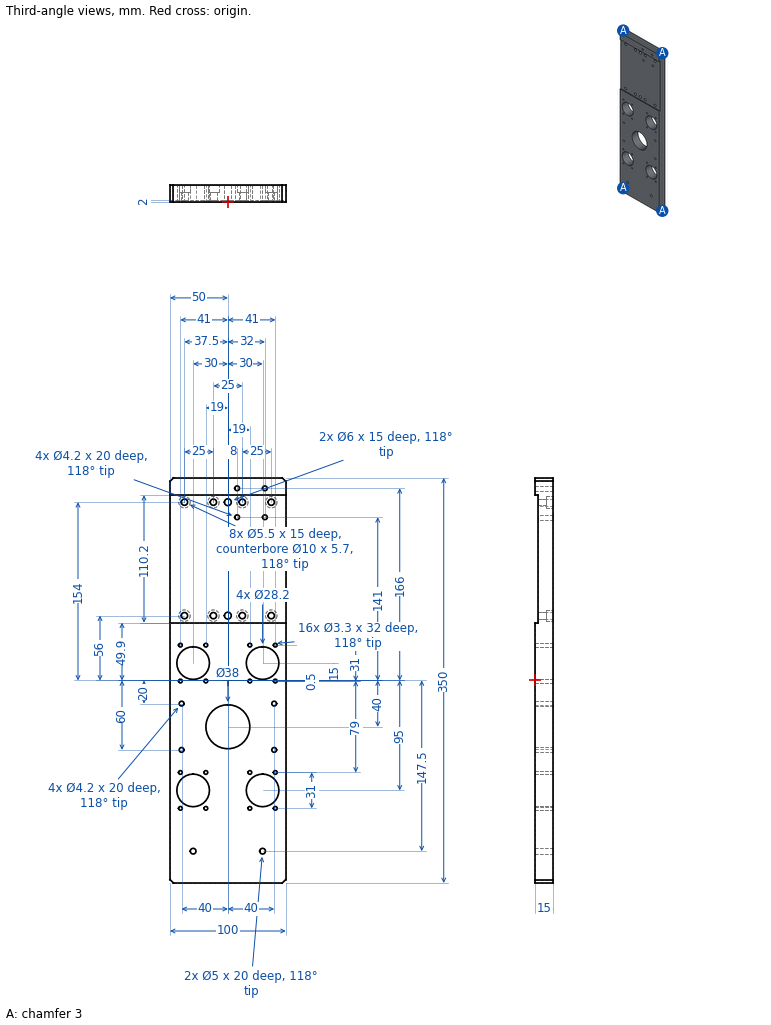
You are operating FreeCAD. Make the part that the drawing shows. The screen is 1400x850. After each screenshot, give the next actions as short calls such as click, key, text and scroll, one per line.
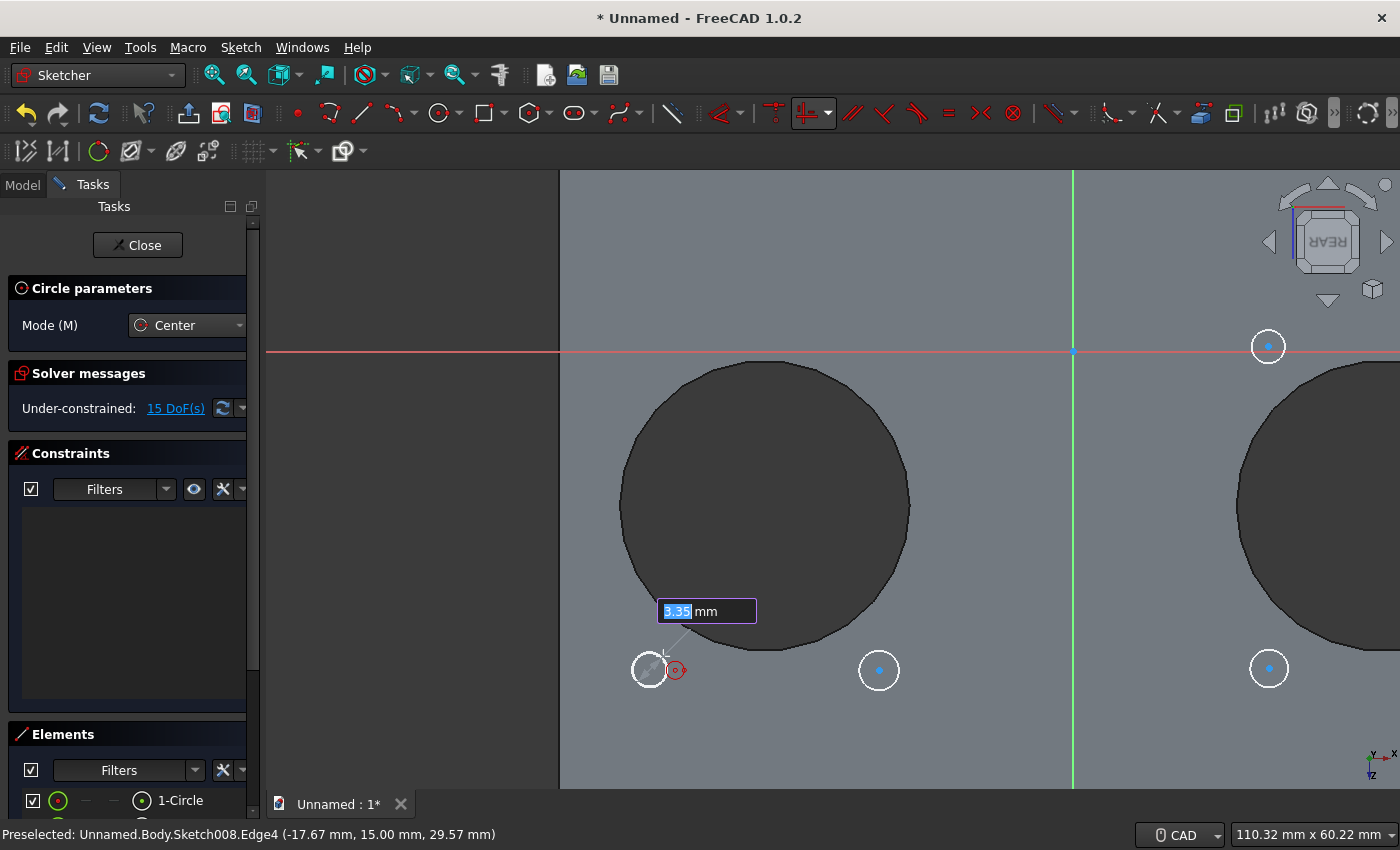
click(664, 653)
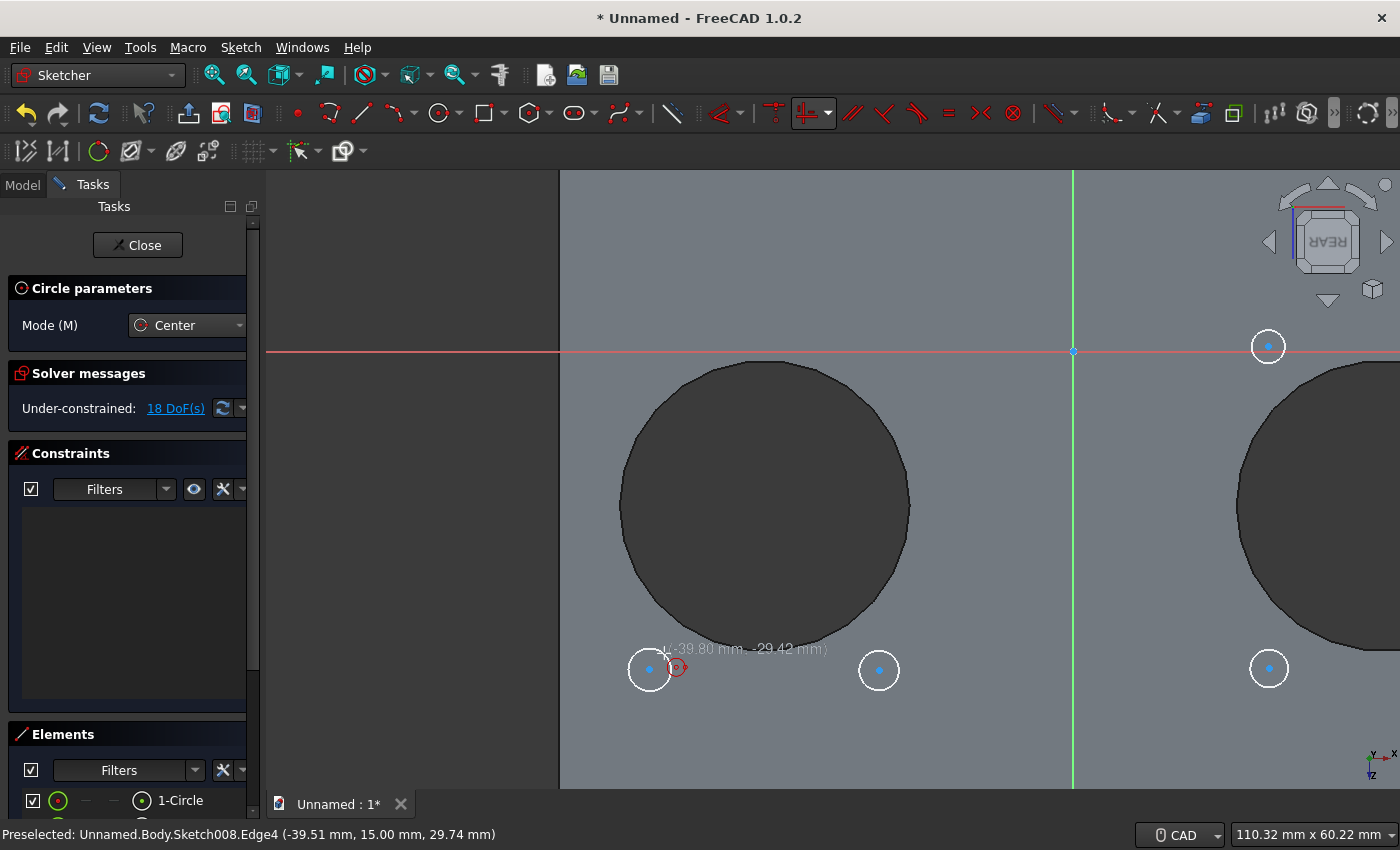
scroll(878, 346, up, 6)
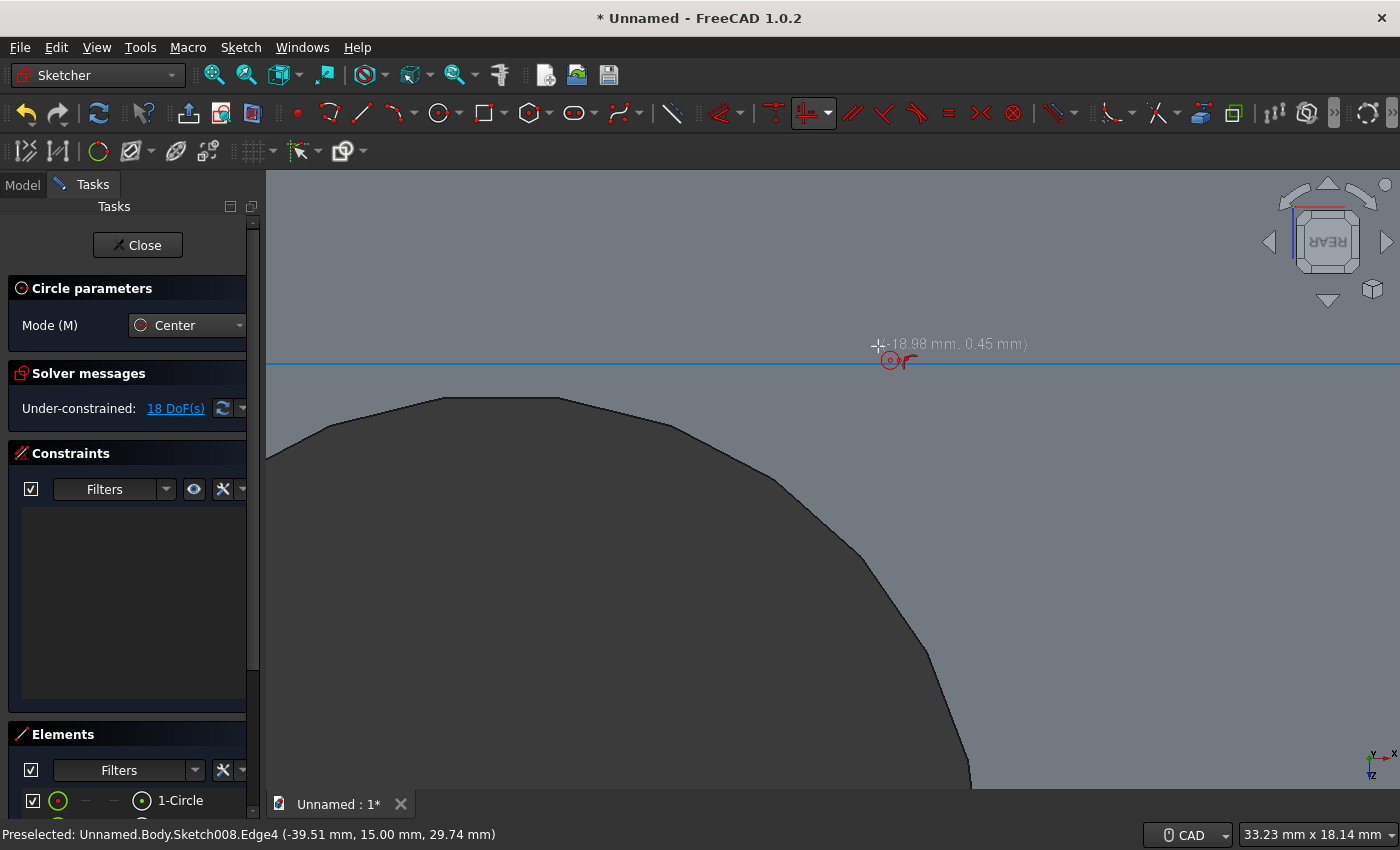
click(876, 347)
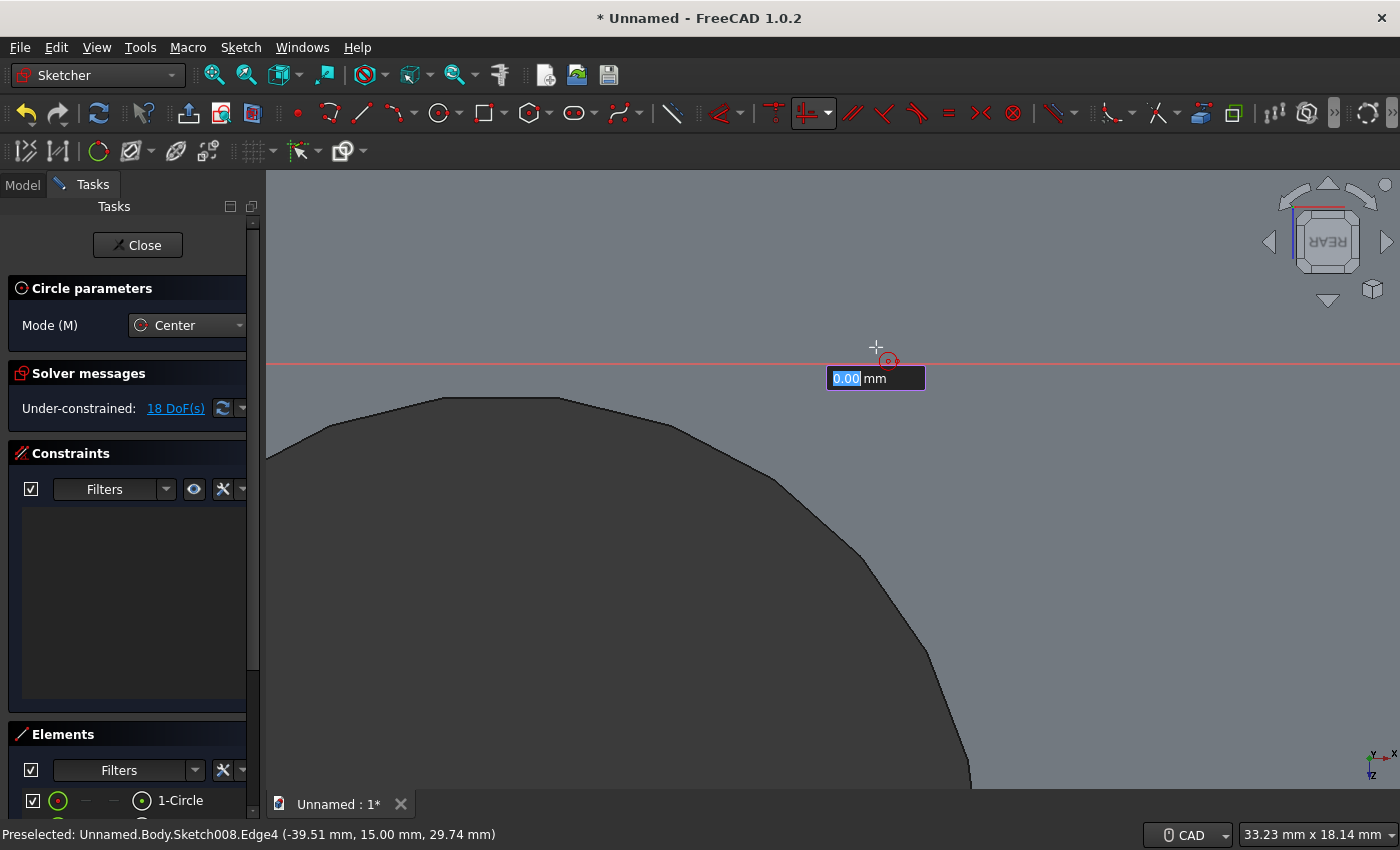
scroll(704, 598, down, 13)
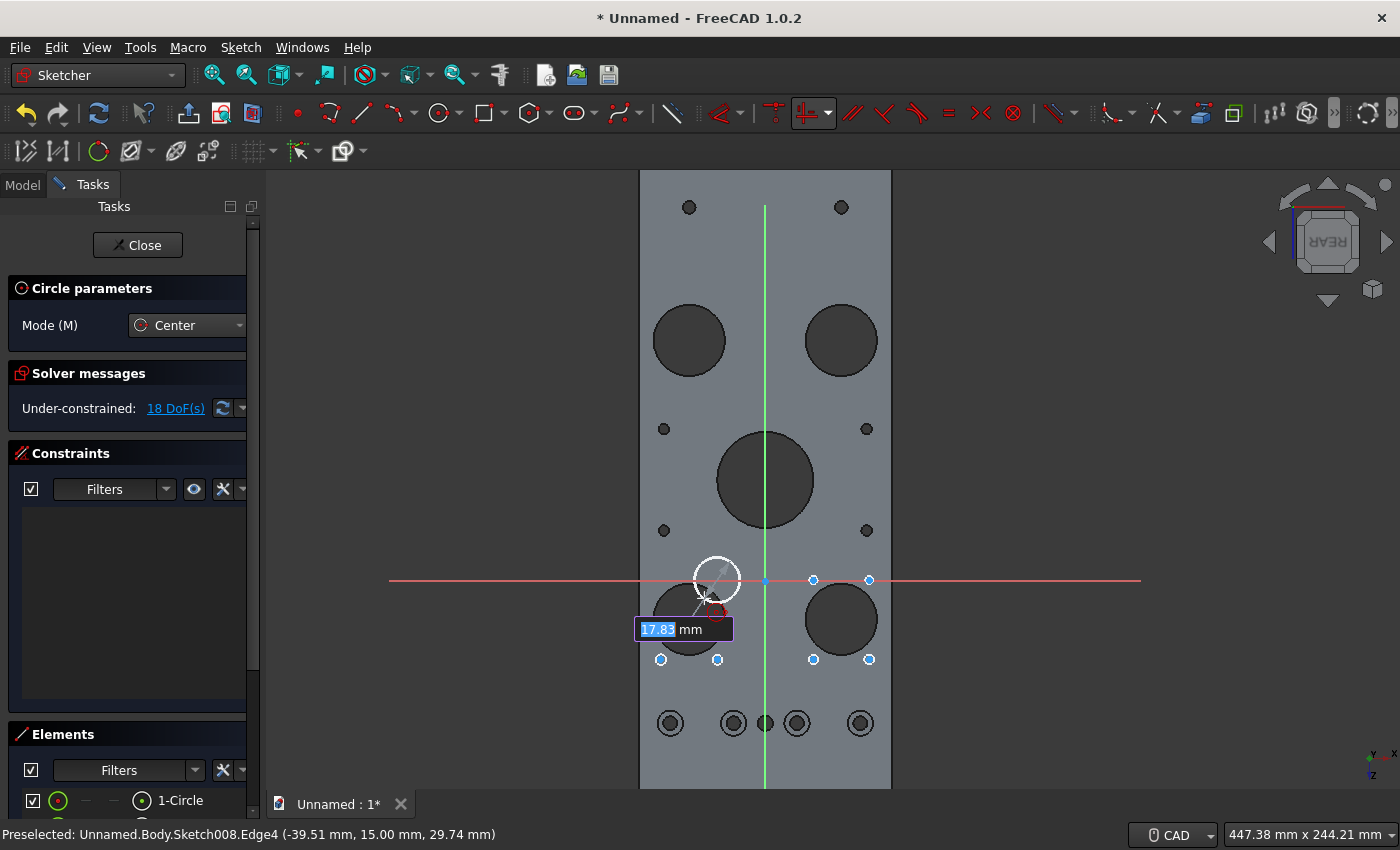
scroll(720, 577, up, 7)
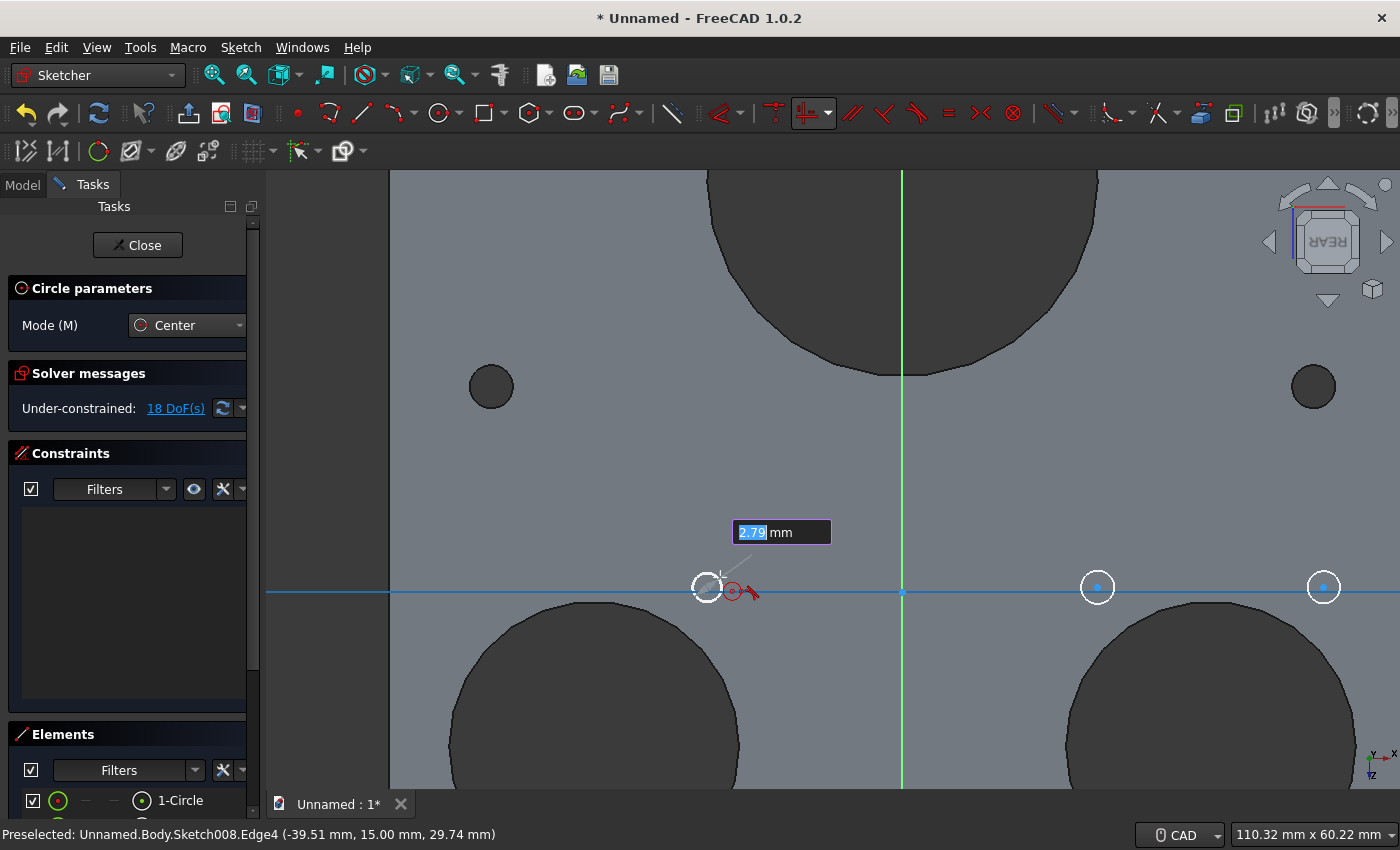
click(719, 575)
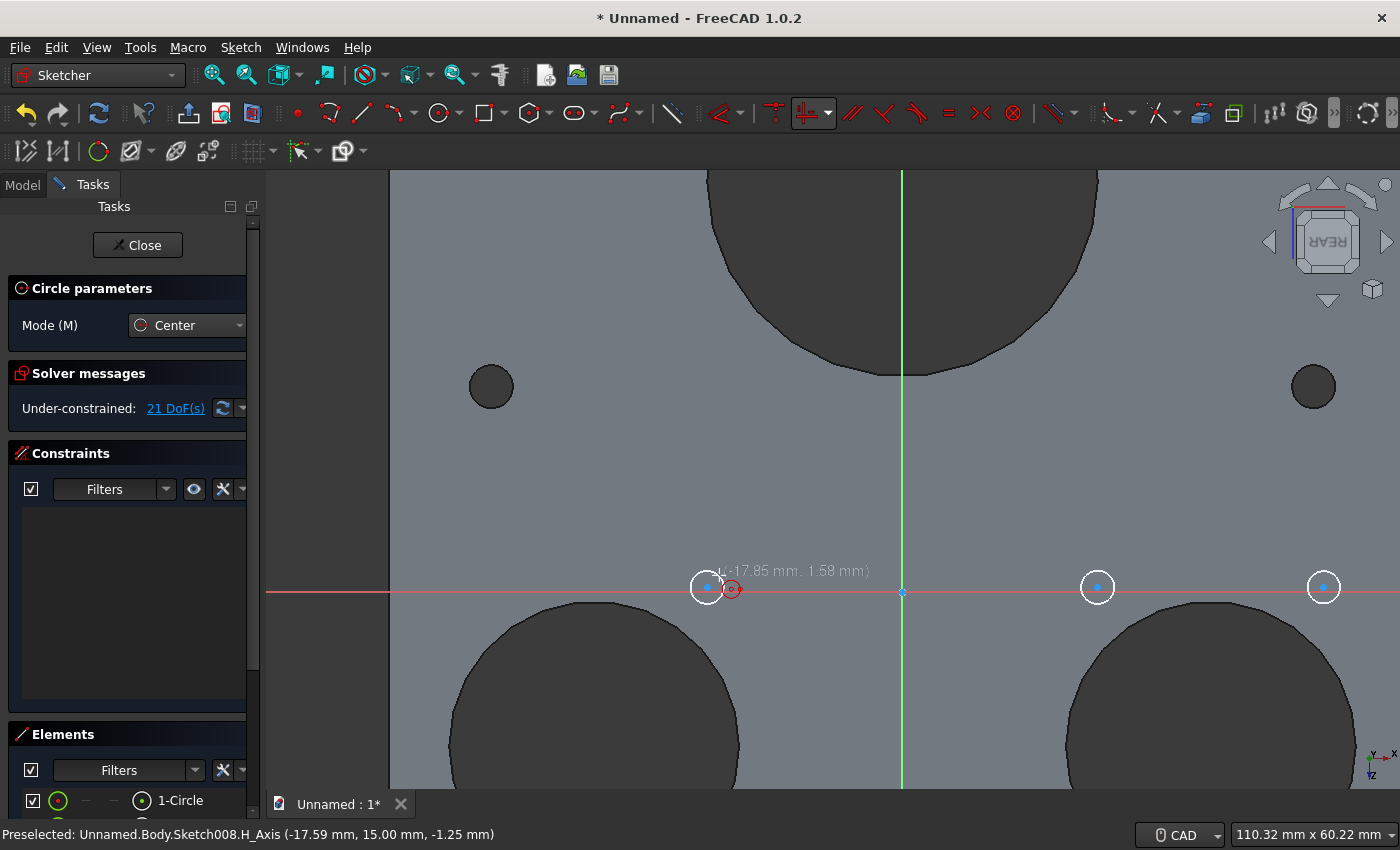
scroll(481, 587, up, 6)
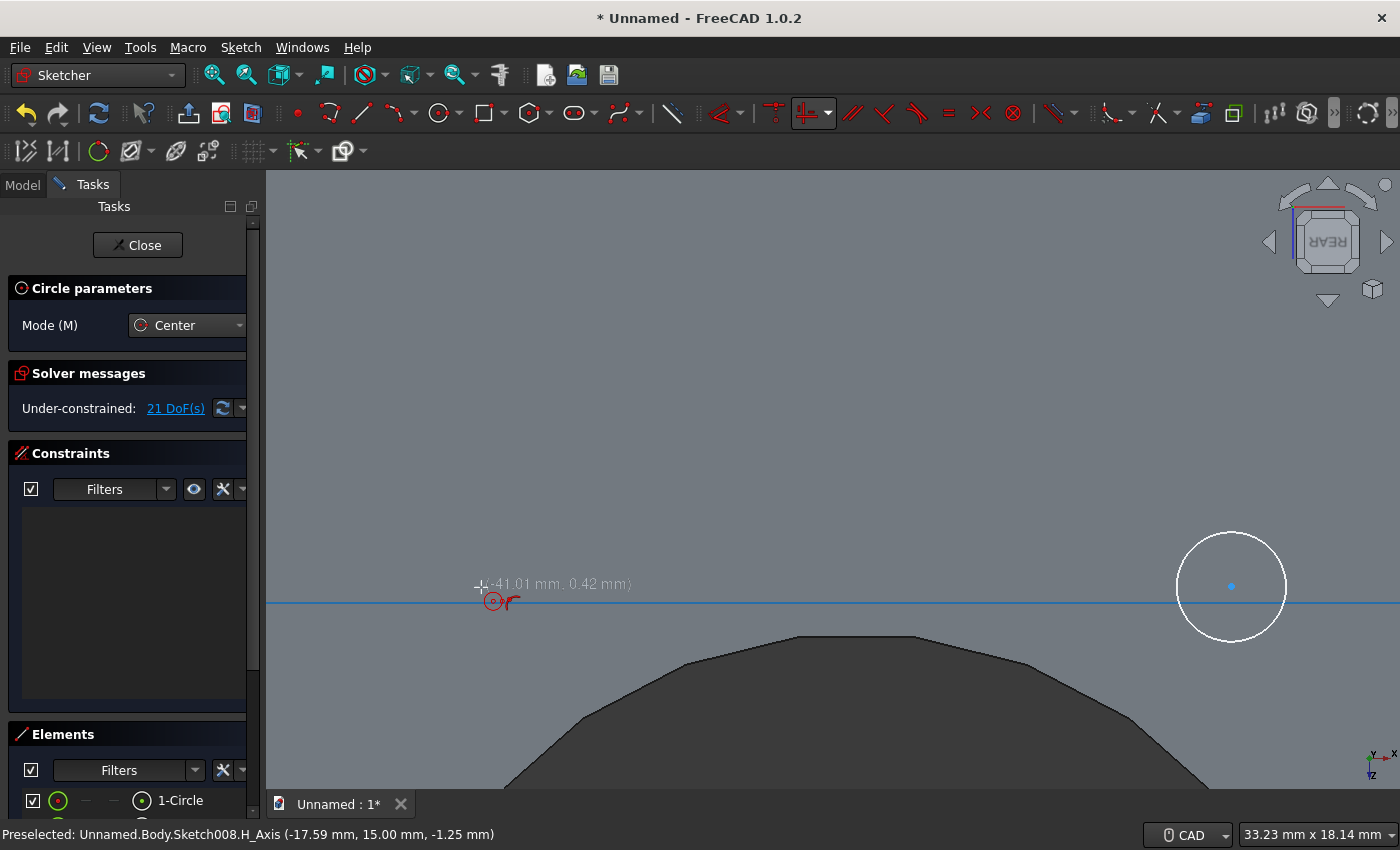
click(481, 586)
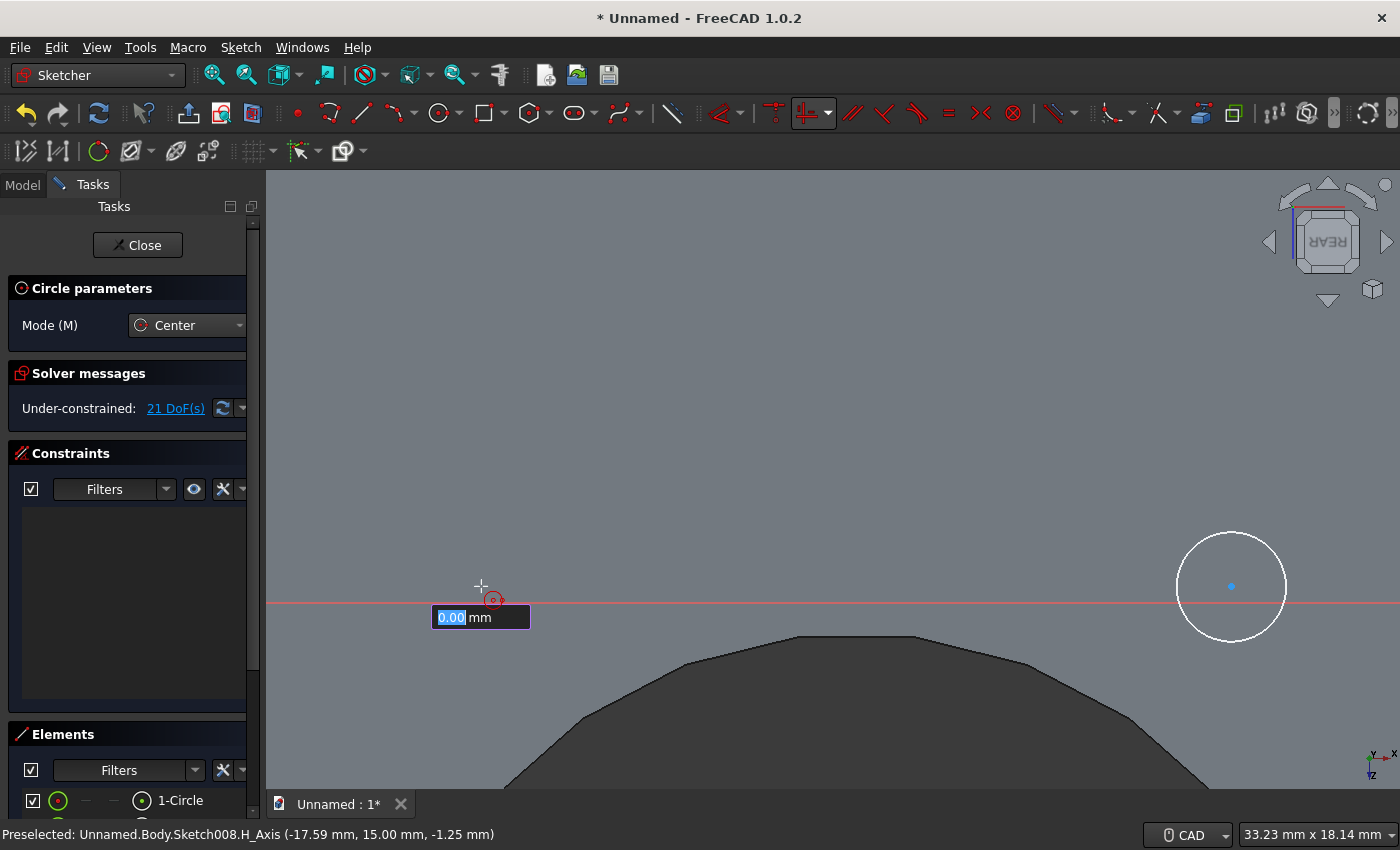
scroll(675, 579, down, 13)